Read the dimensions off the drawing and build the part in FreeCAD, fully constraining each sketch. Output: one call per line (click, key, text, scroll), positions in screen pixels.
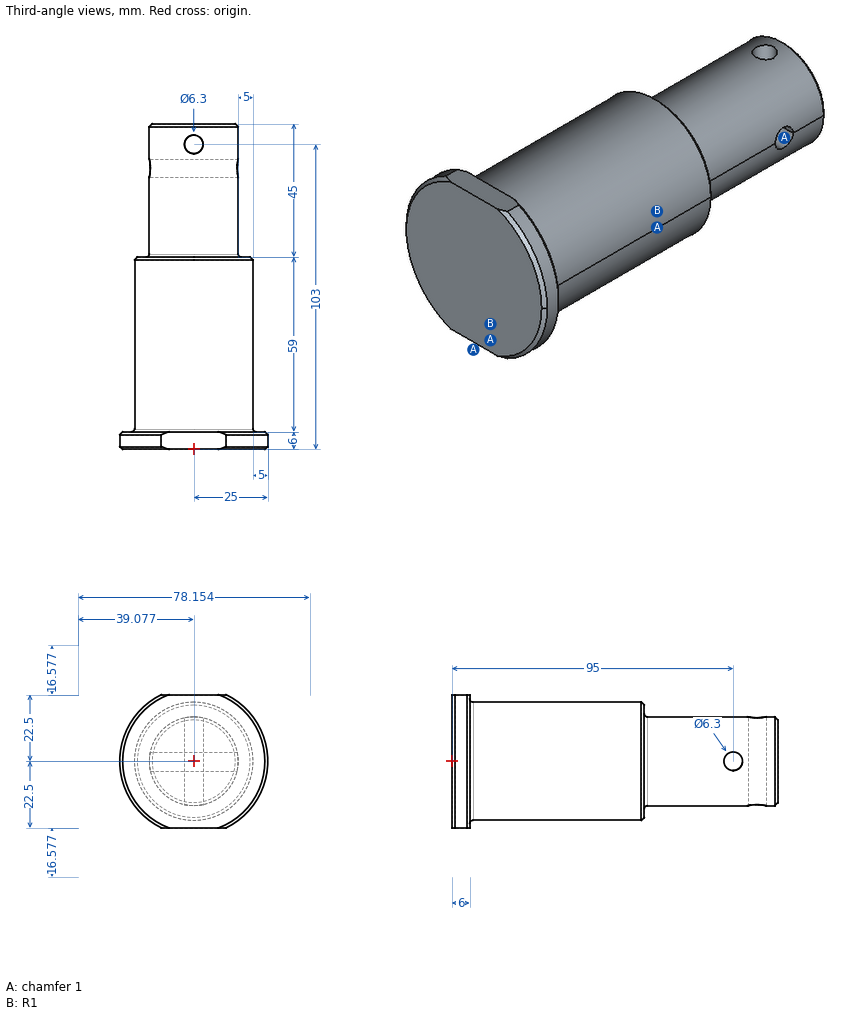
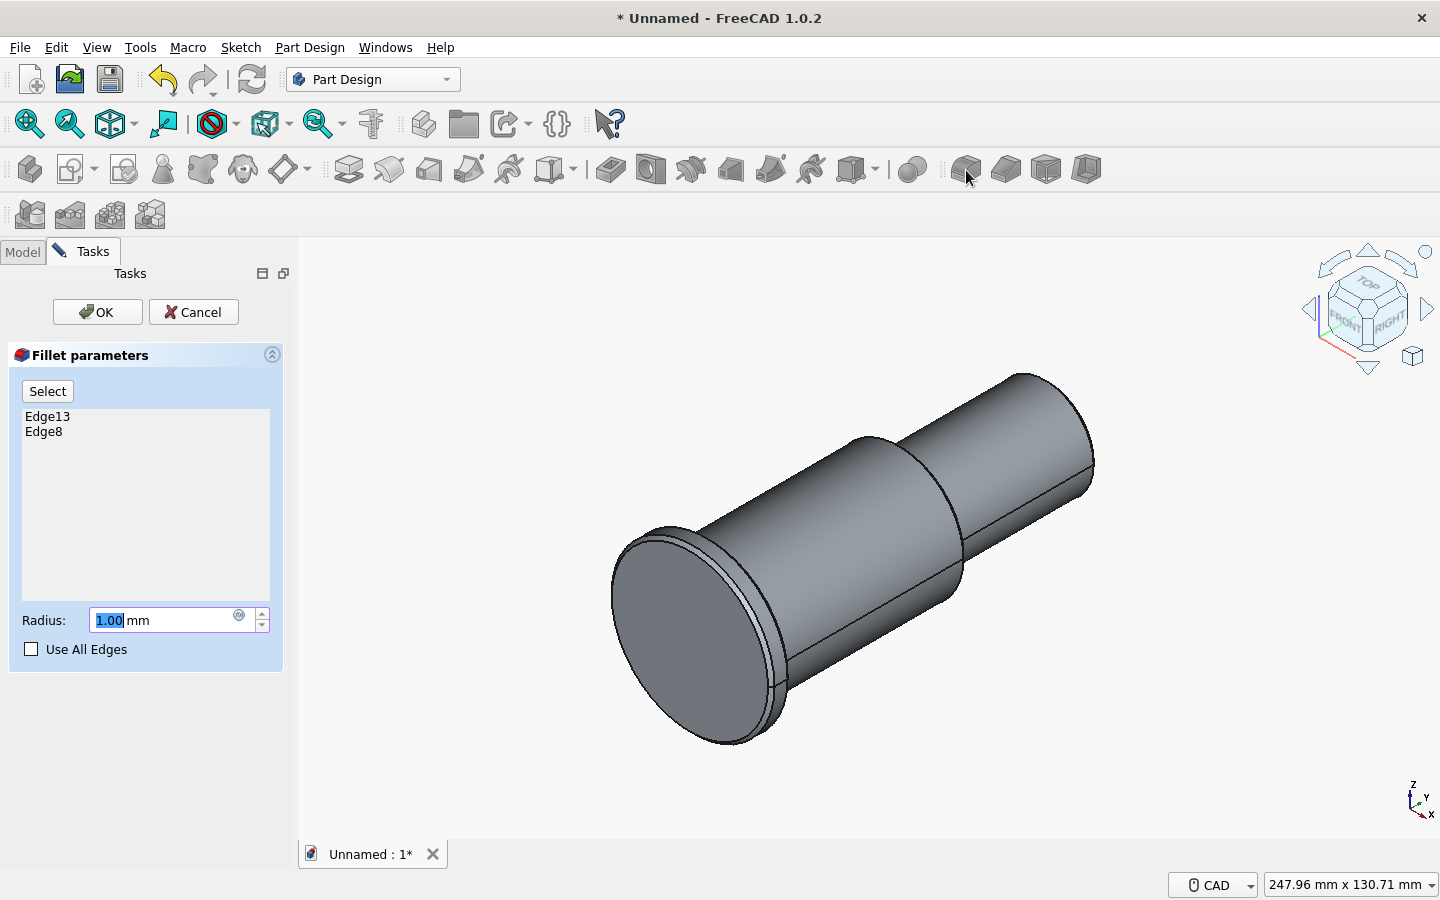
text(1)
key(Tab)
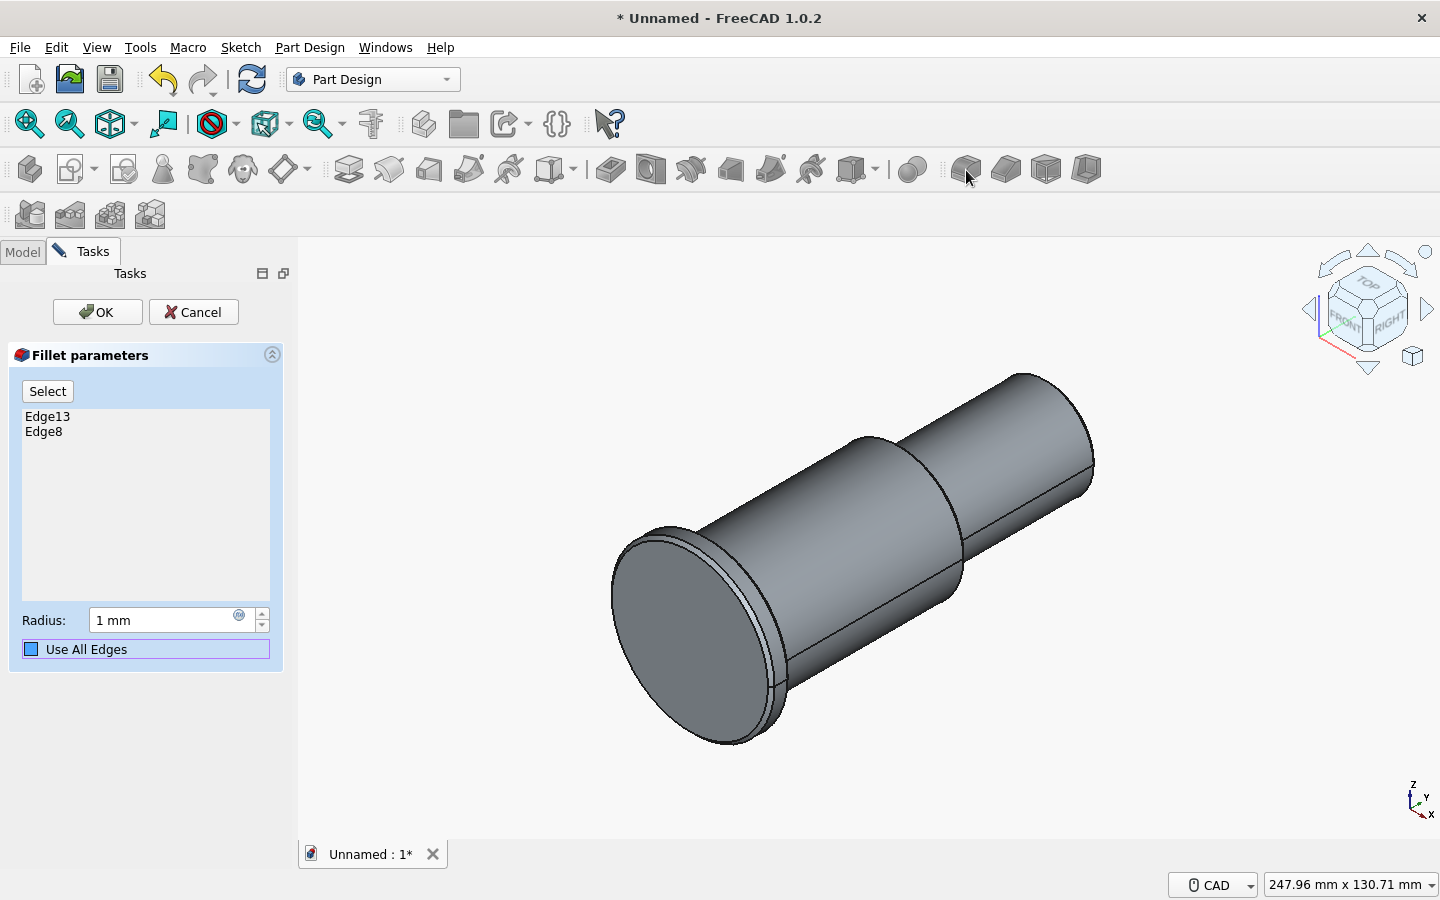
click(98, 312)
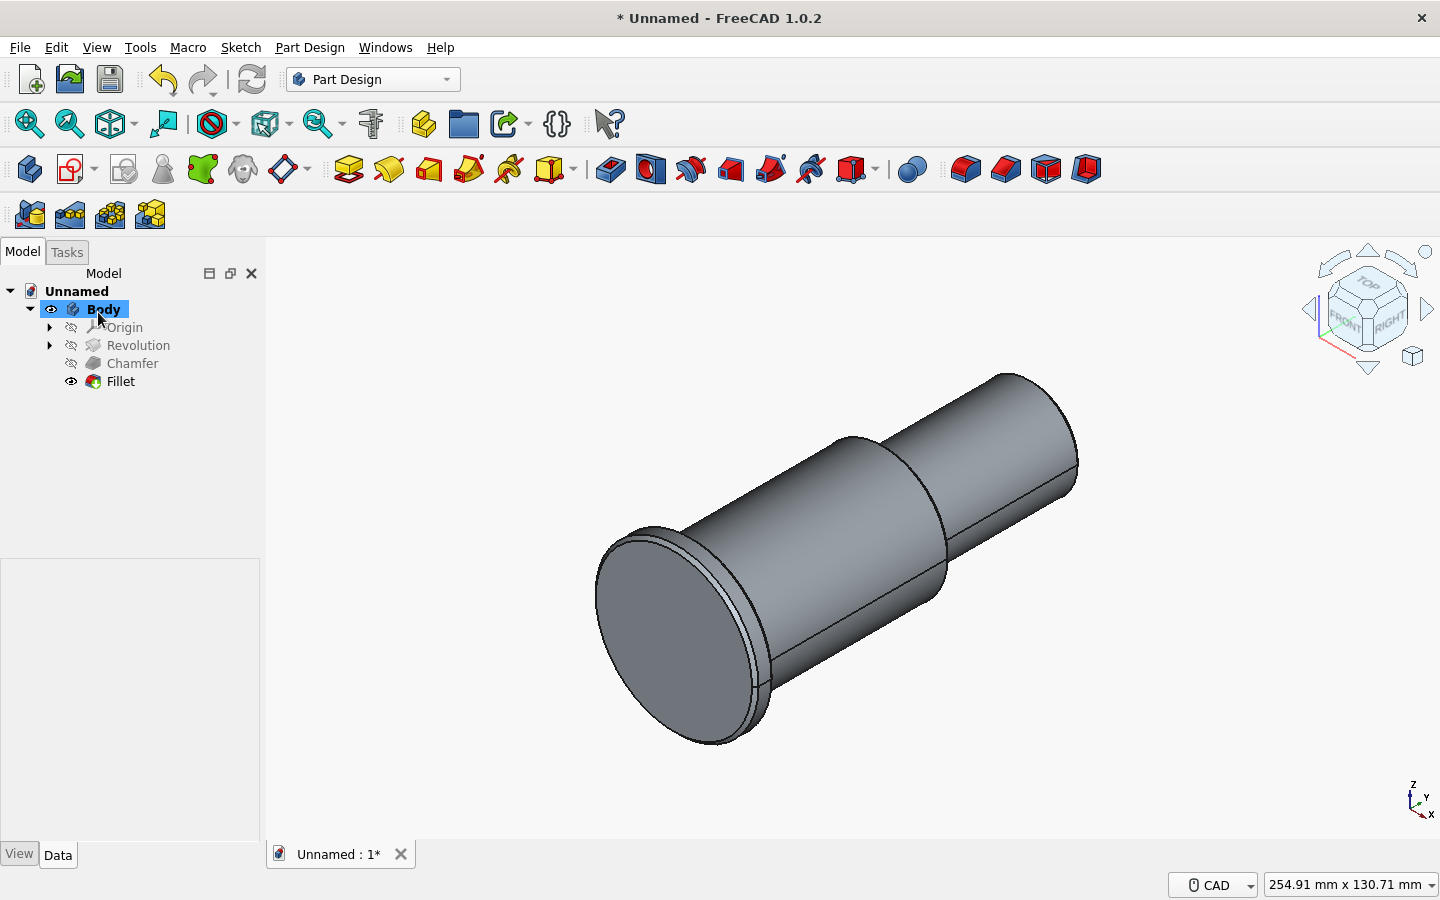
click(674, 640)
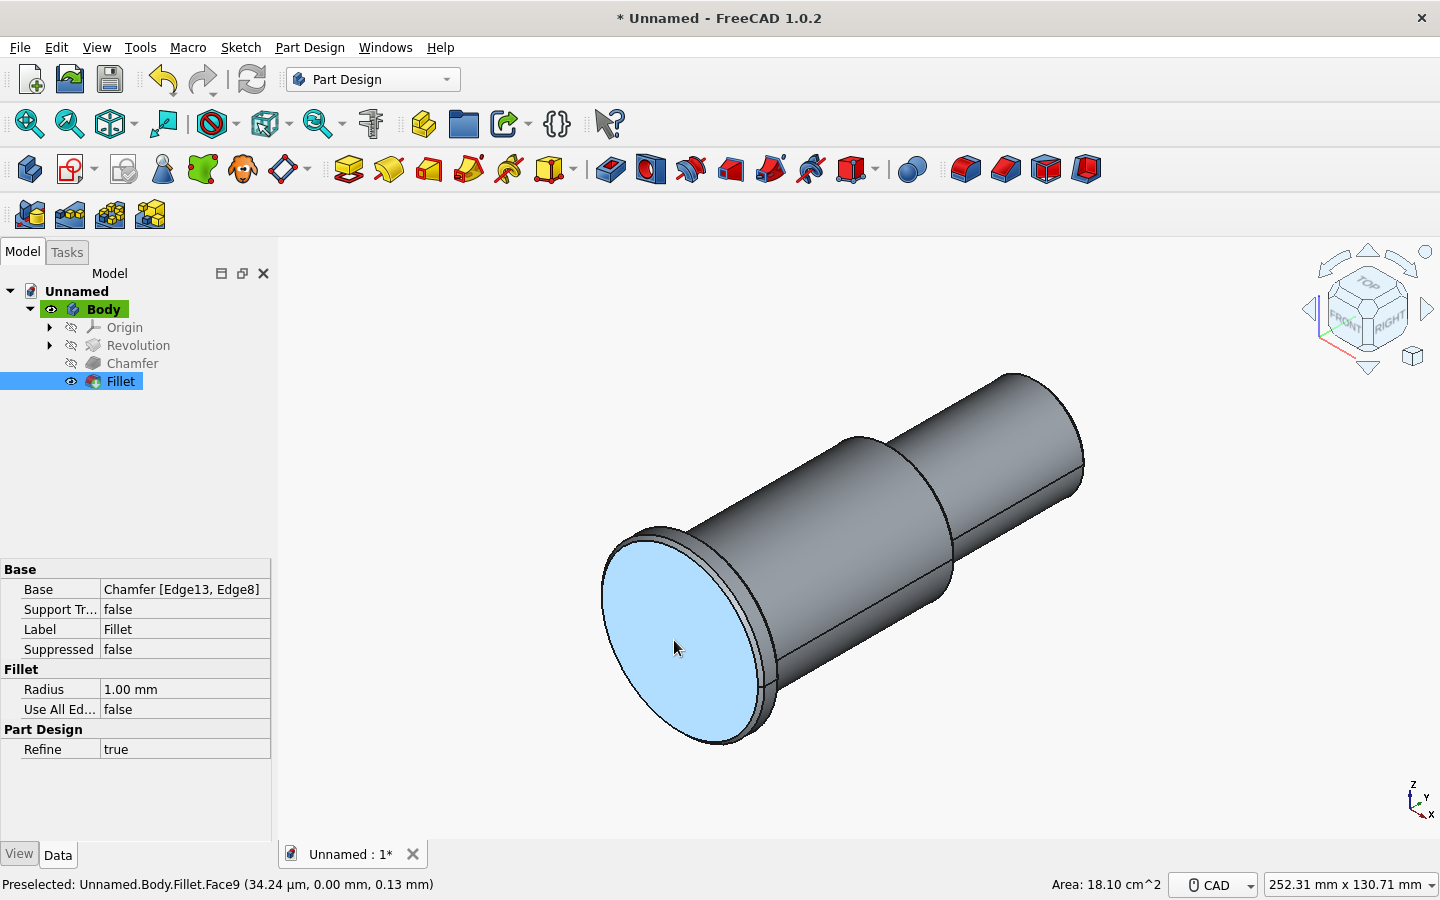
click(70, 170)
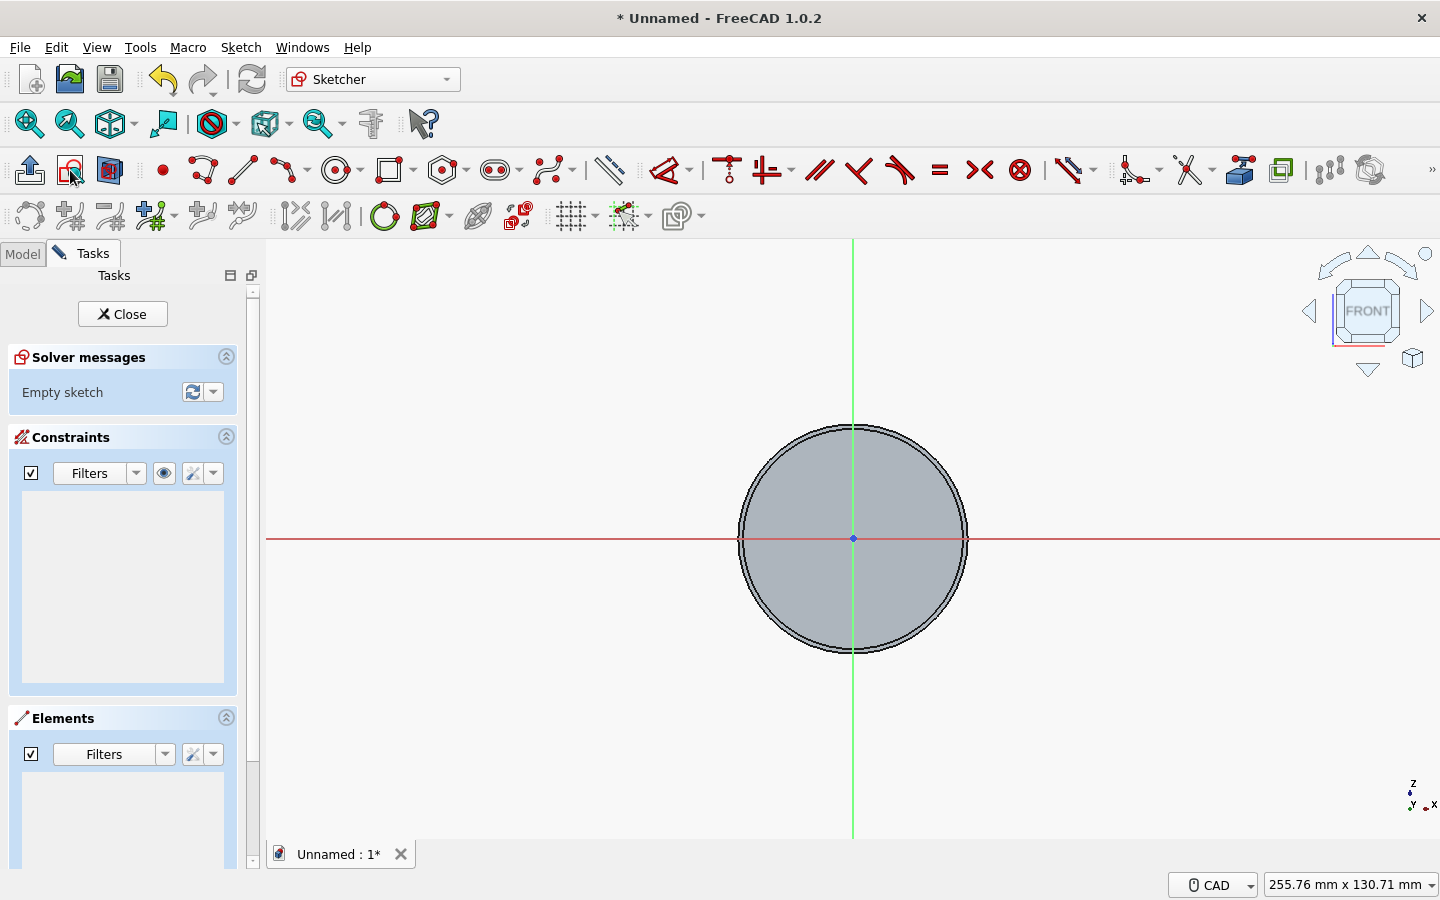
click(390, 170)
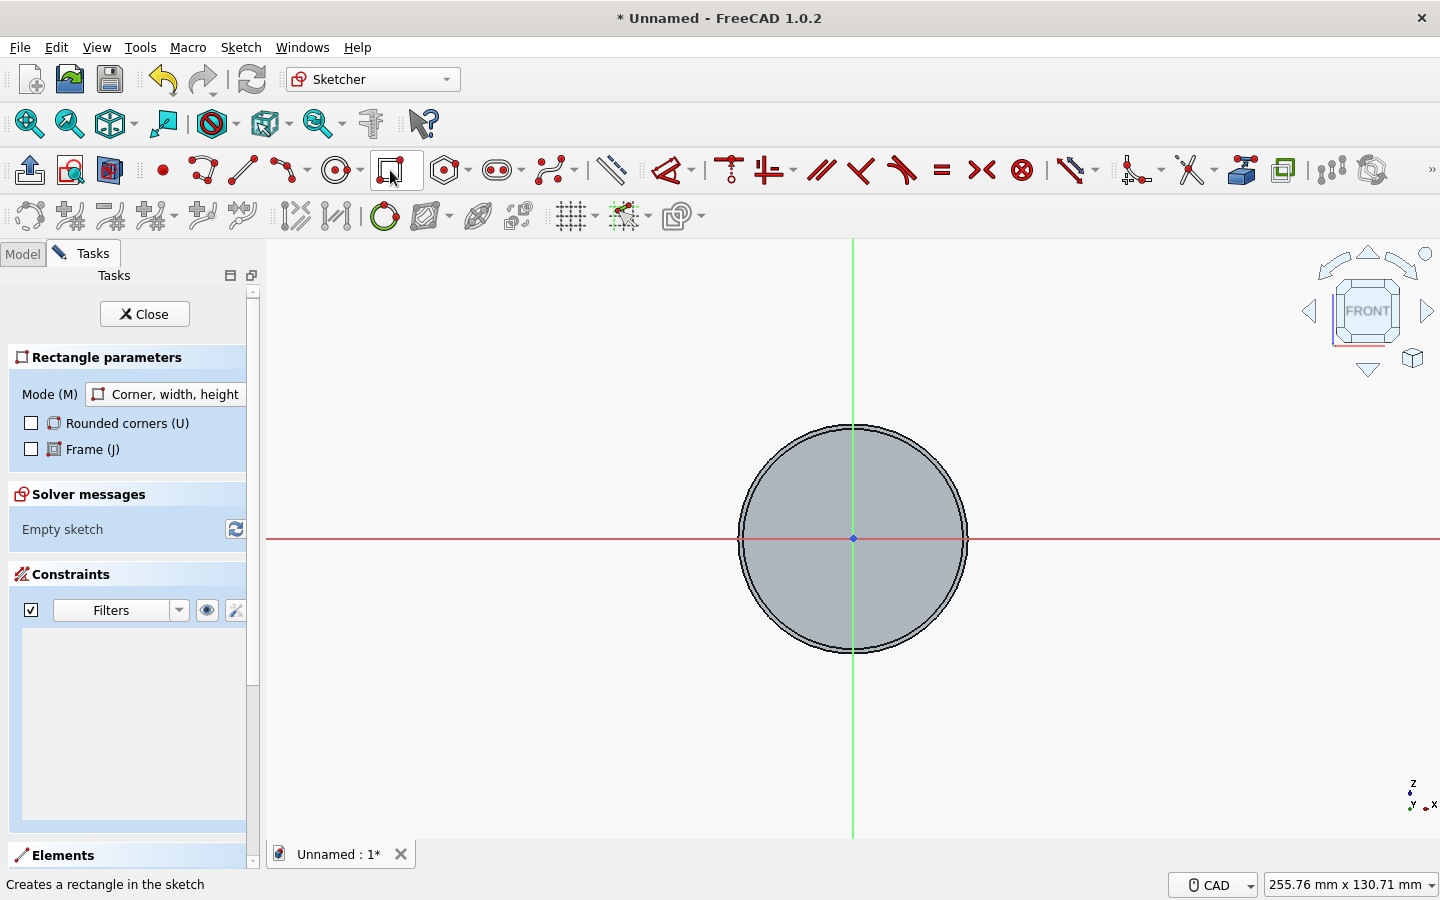
click(674, 360)
click(1032, 436)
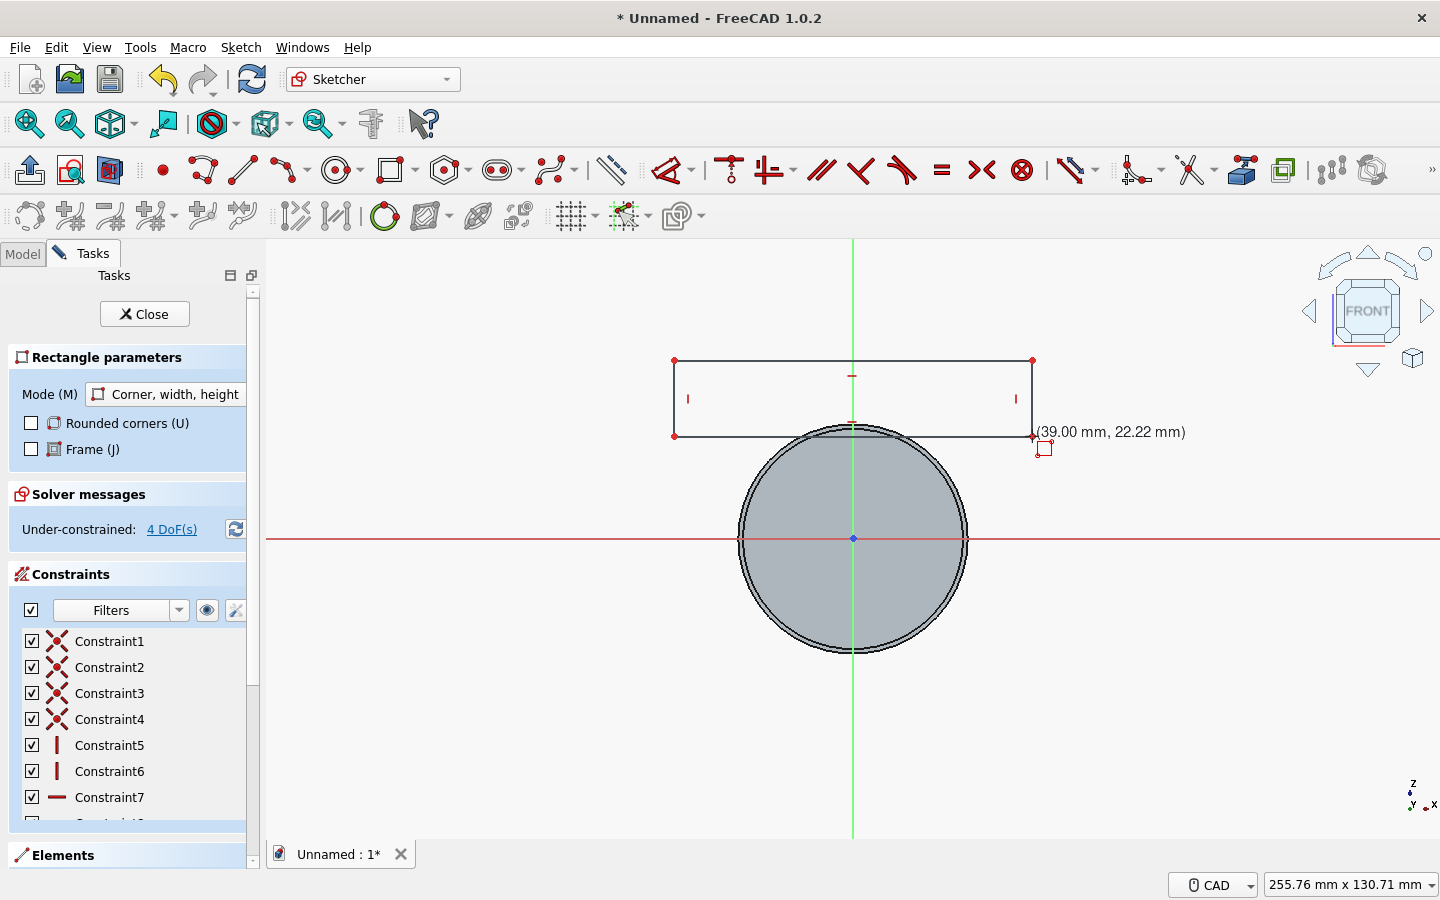
click(674, 642)
click(1032, 718)
key(Escape)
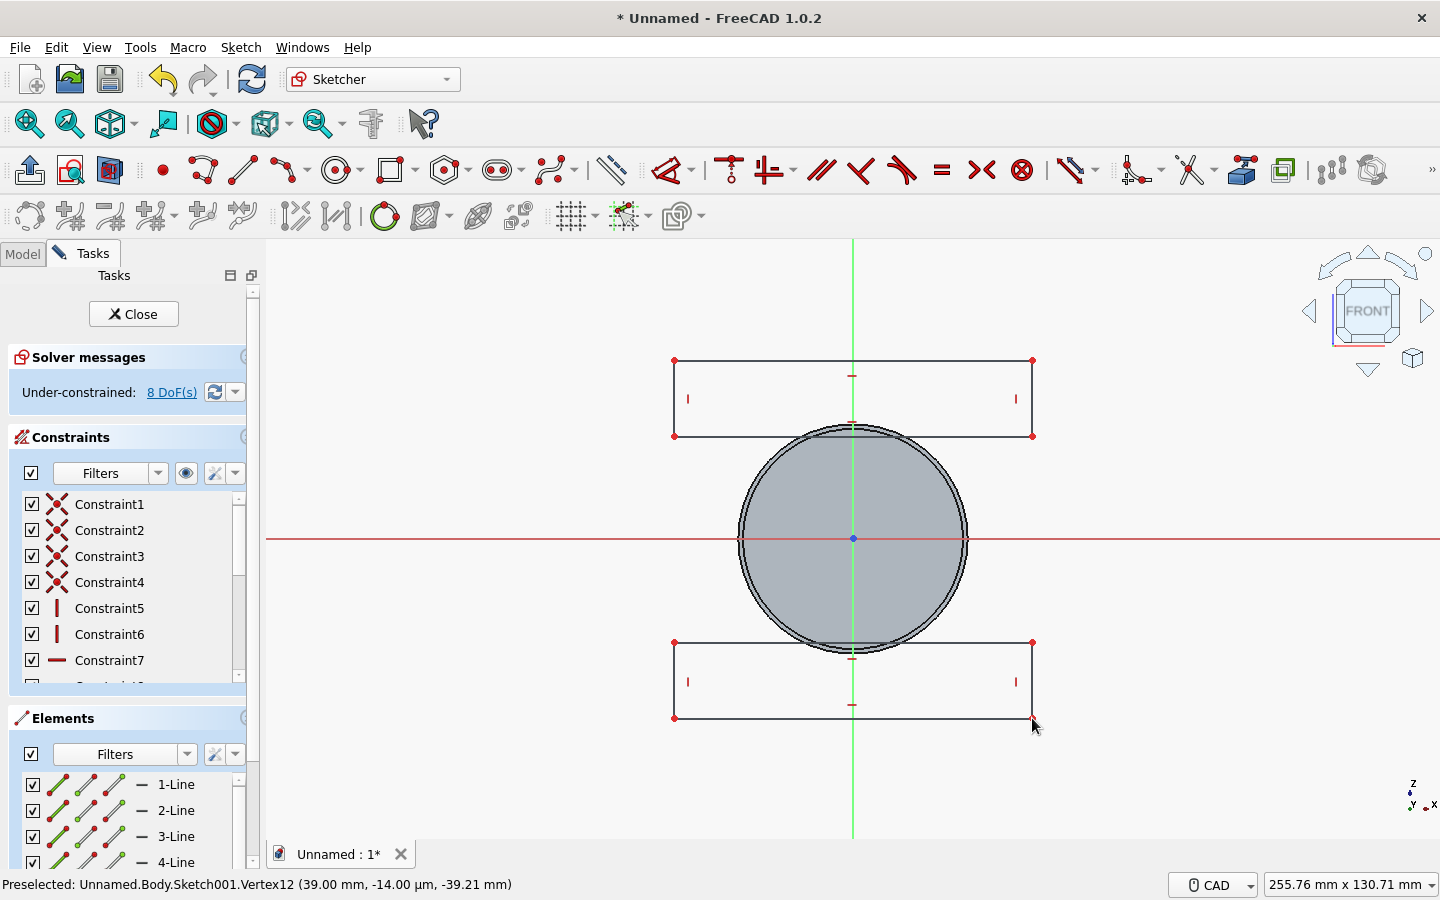
key(d)